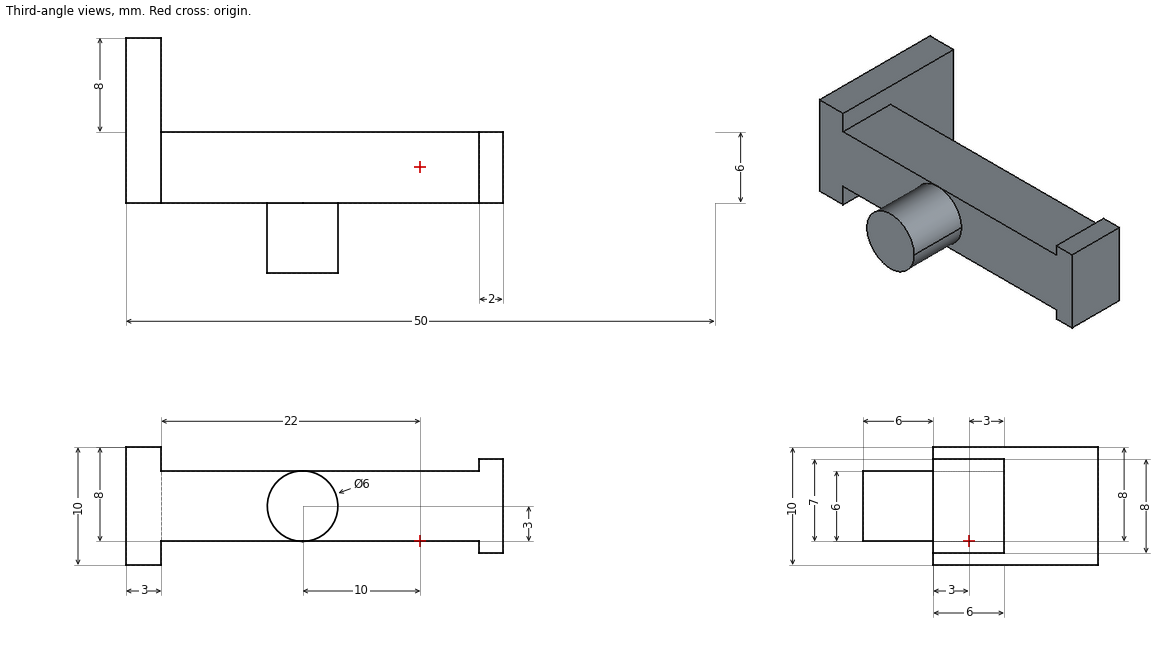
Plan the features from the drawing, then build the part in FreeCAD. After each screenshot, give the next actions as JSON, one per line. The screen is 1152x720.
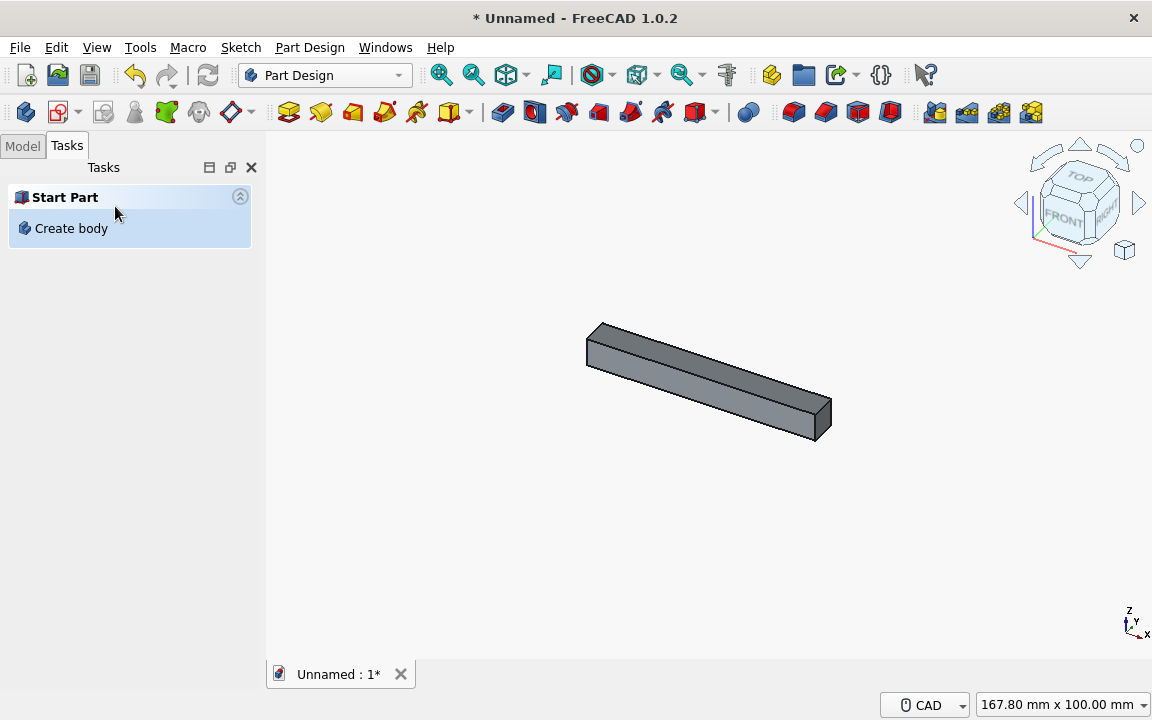
{"action": "left_click", "coordinate": [442, 76]}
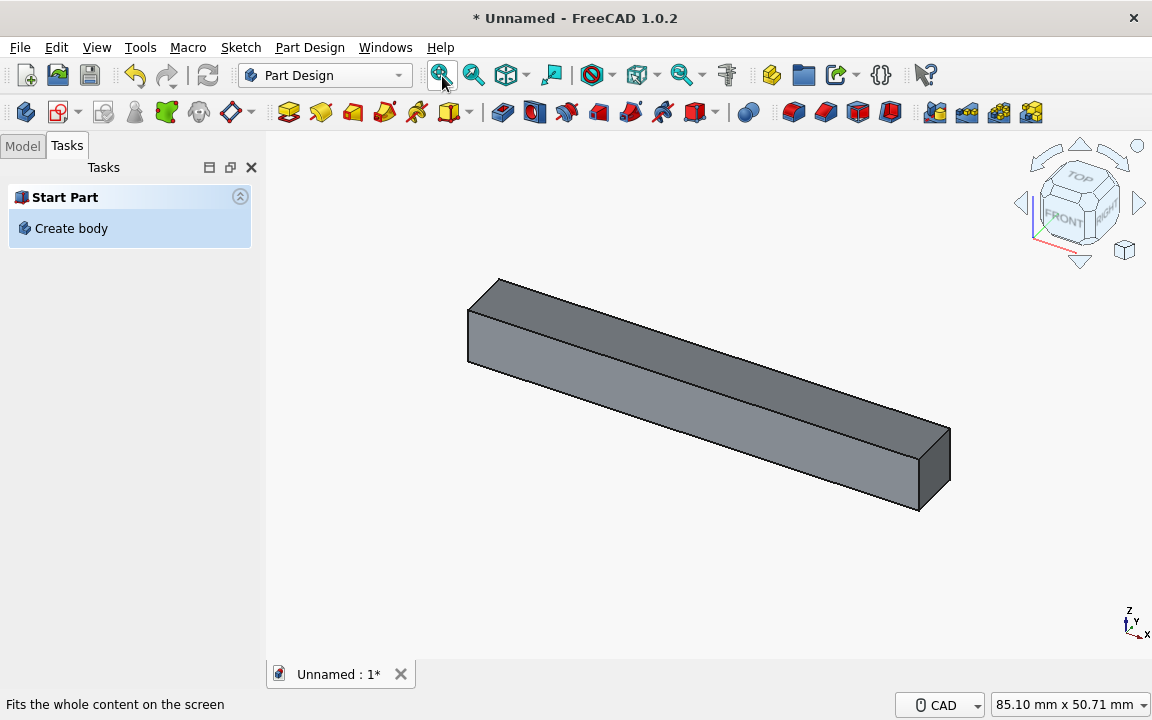
{"action": "left_click", "coordinate": [887, 473]}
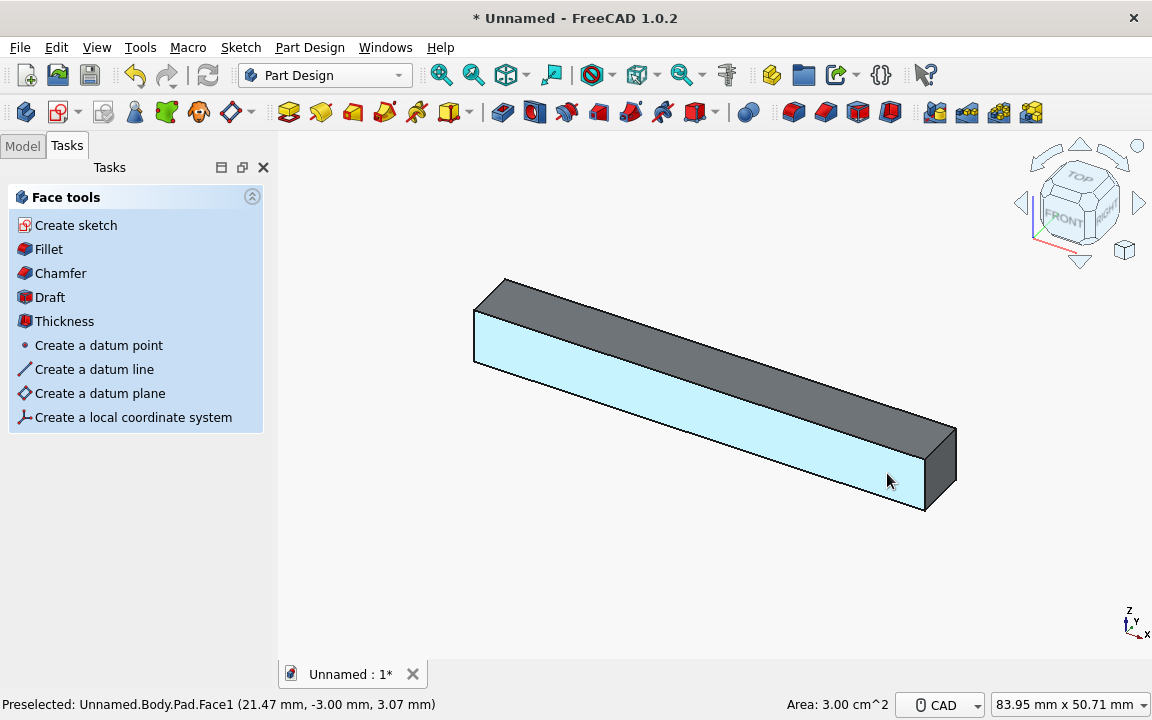
{"action": "left_click", "coordinate": [58, 112]}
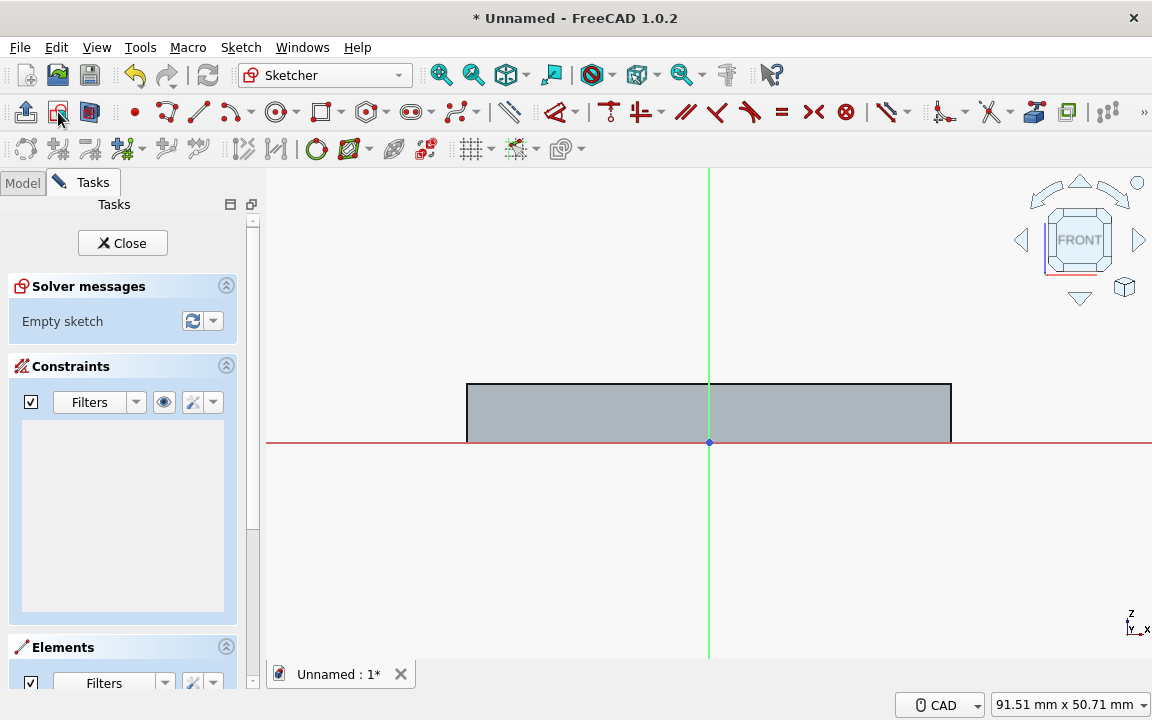
{"action": "scroll", "coordinate": [648, 414], "scroll_direction": "up", "scroll_amount": 7}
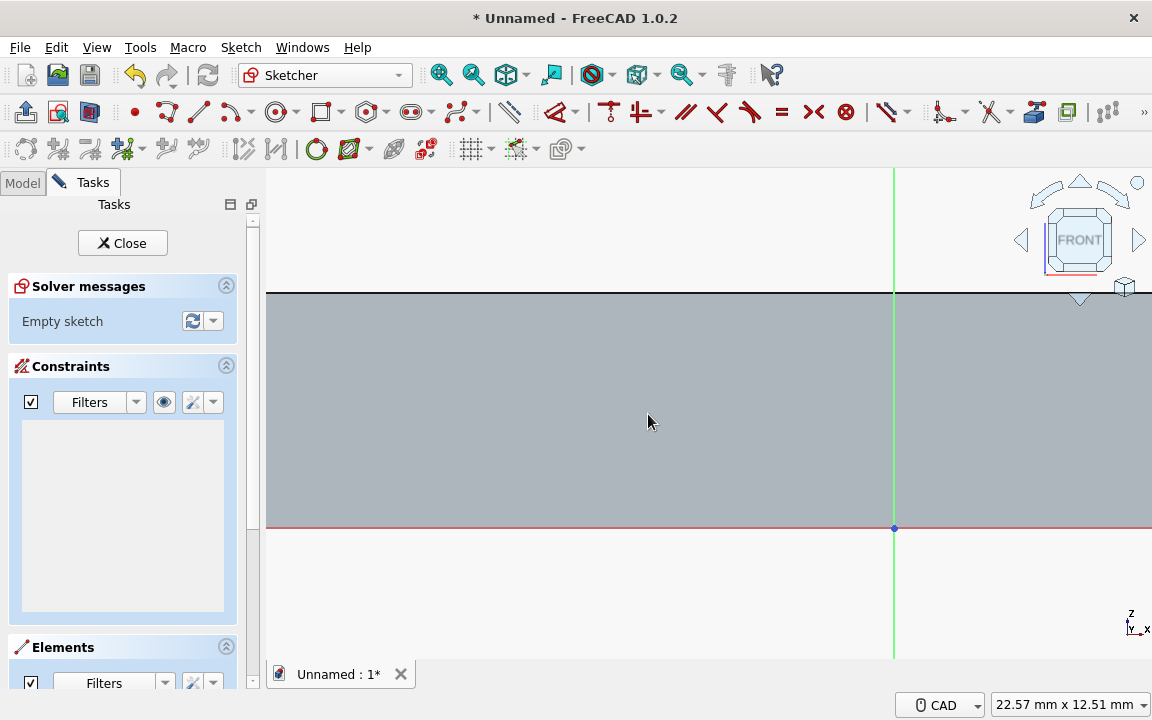
{"action": "left_click", "coordinate": [276, 112]}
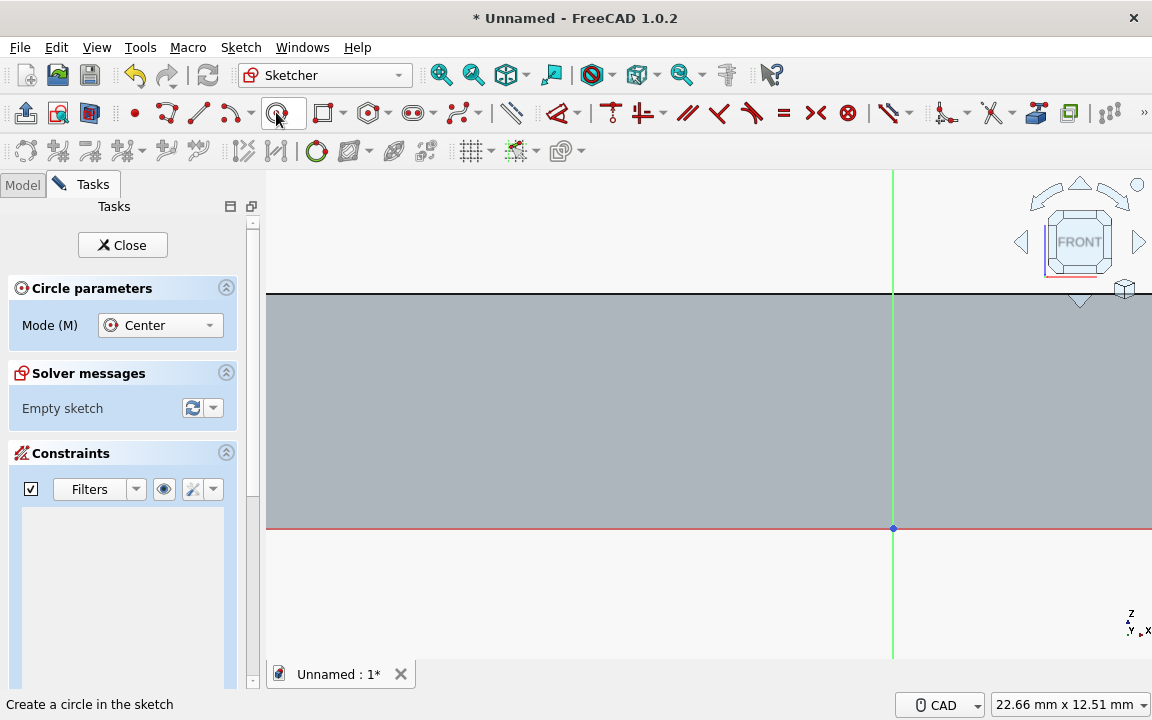
{"action": "left_click", "coordinate": [502, 411]}
{"action": "mouse_move", "coordinate": [585, 329]}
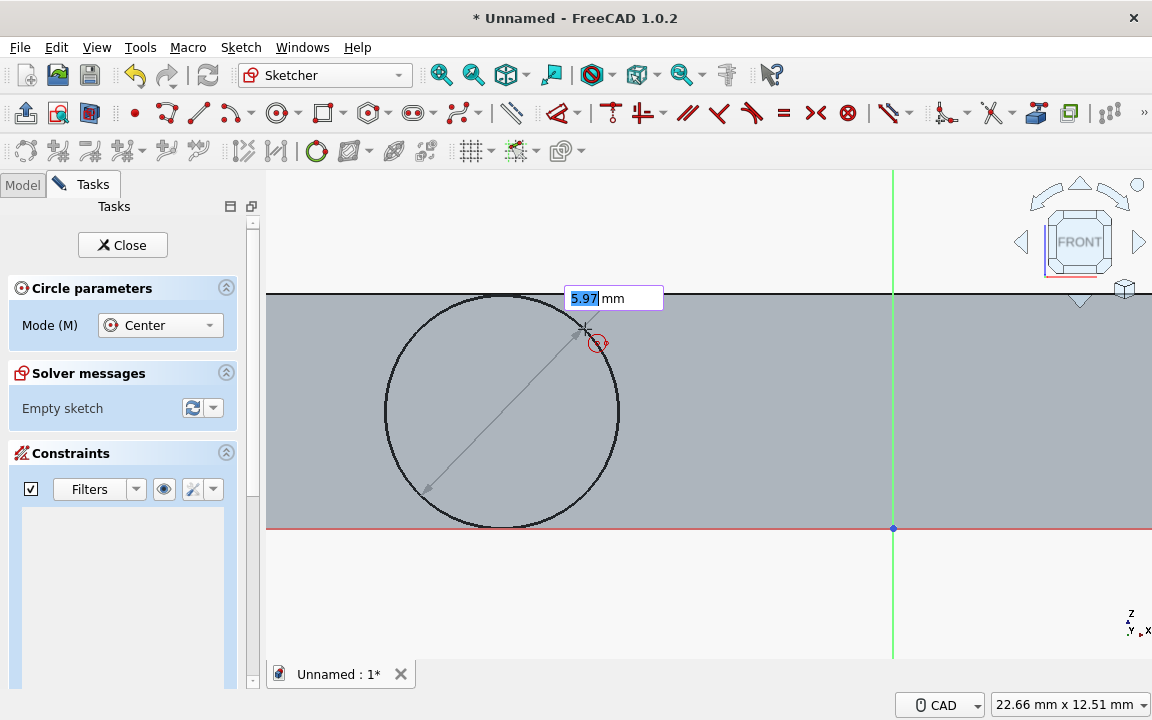
{"action": "type", "text": "6"}
{"action": "key", "text": "Return"}
{"action": "key", "text": "Escape"}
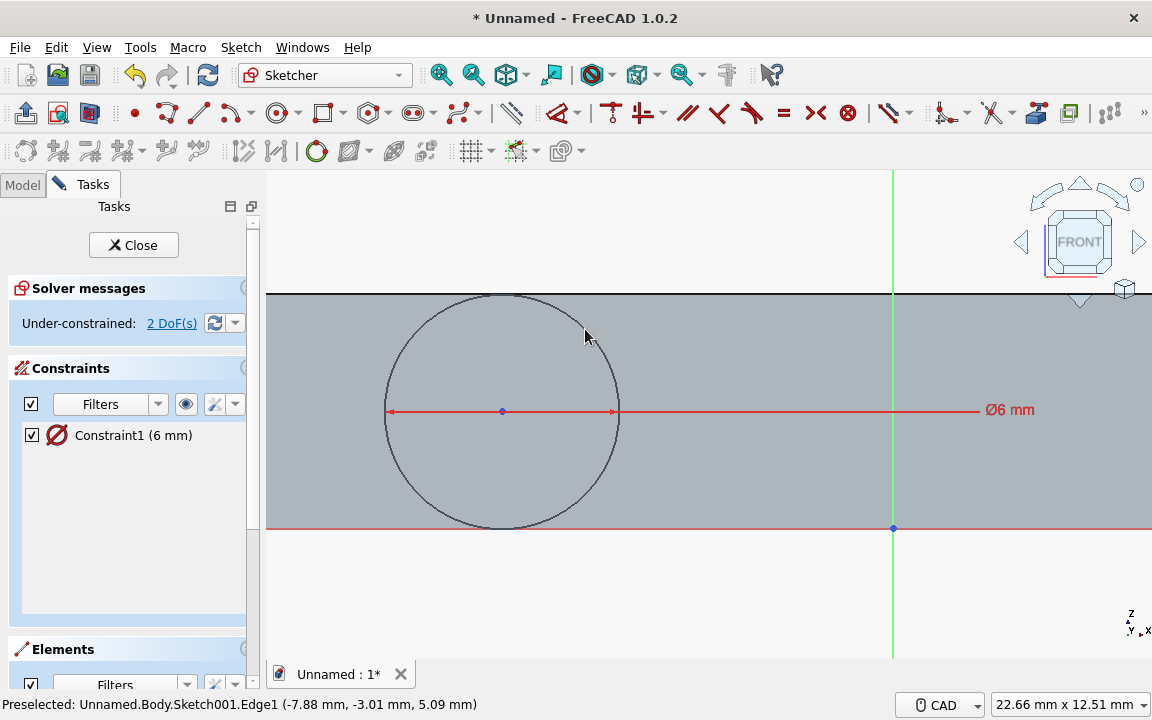
{"action": "left_click", "coordinate": [558, 114]}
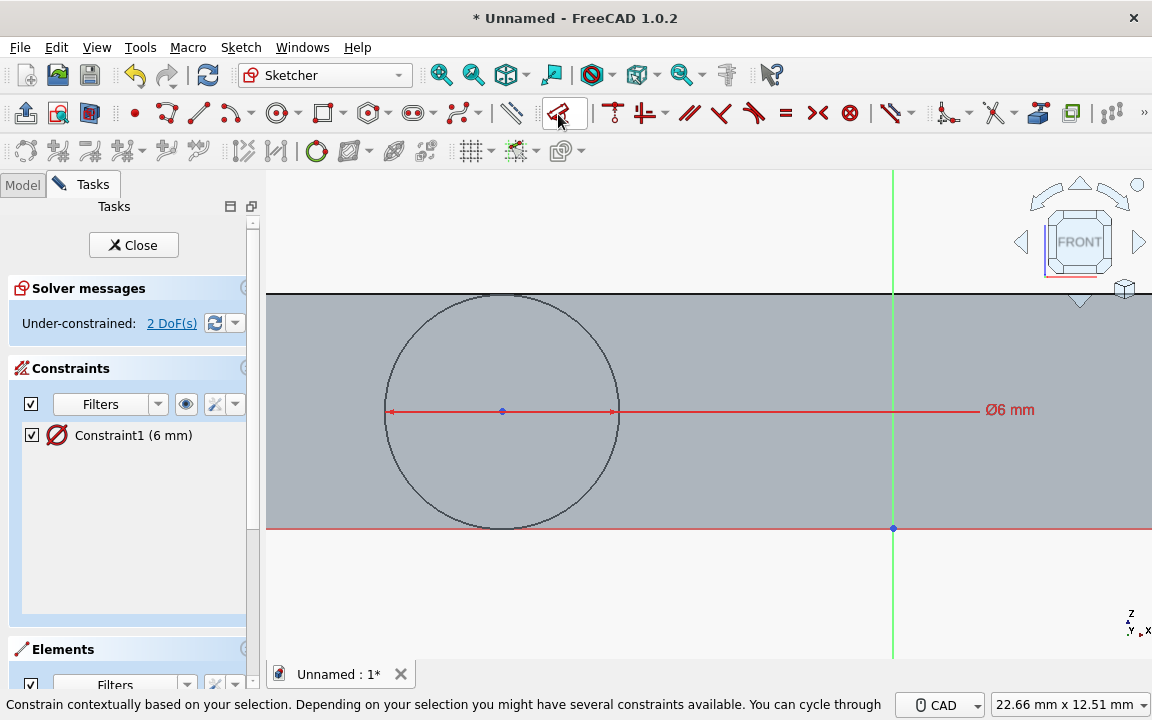
{"action": "left_click", "coordinate": [502, 412]}
{"action": "left_click", "coordinate": [927, 470]}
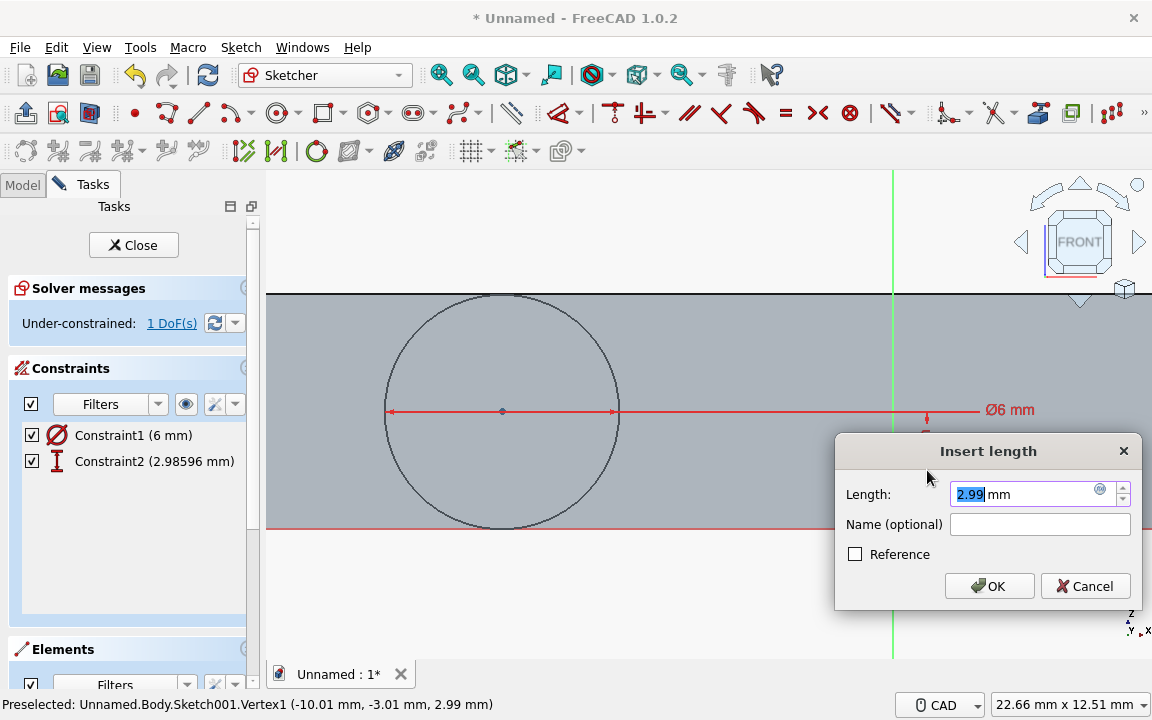
{"action": "type", "text": "3"}
{"action": "key", "text": "Return"}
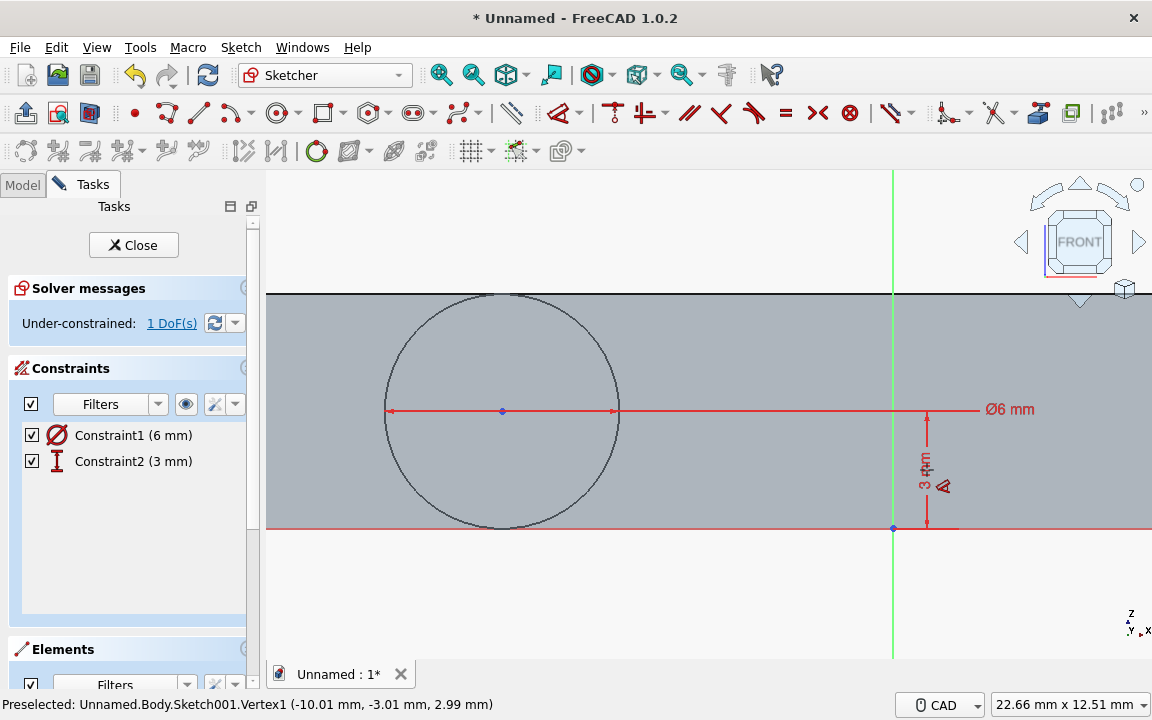
{"action": "left_click", "coordinate": [502, 411]}
{"action": "left_click", "coordinate": [698, 563]}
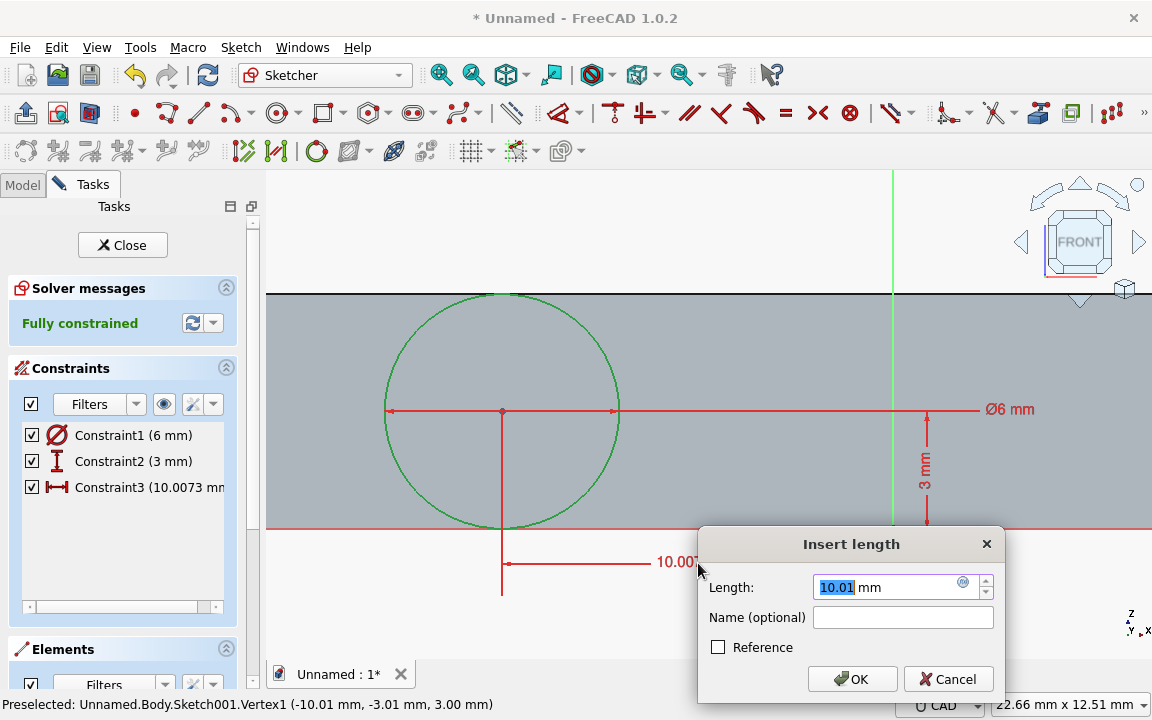
{"action": "type", "text": "10"}
{"action": "key", "text": "Return"}
{"action": "key", "text": "Escape"}